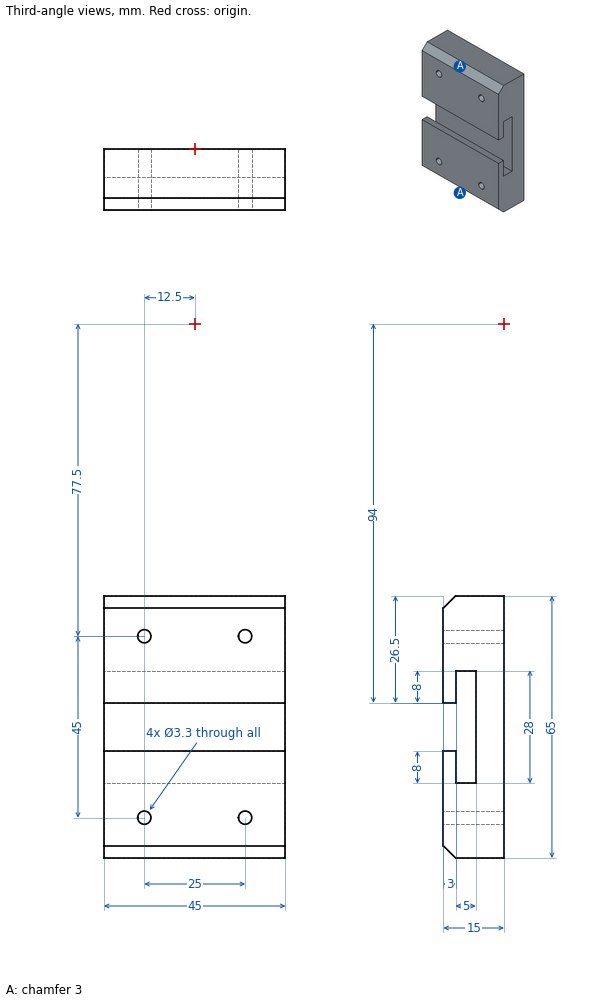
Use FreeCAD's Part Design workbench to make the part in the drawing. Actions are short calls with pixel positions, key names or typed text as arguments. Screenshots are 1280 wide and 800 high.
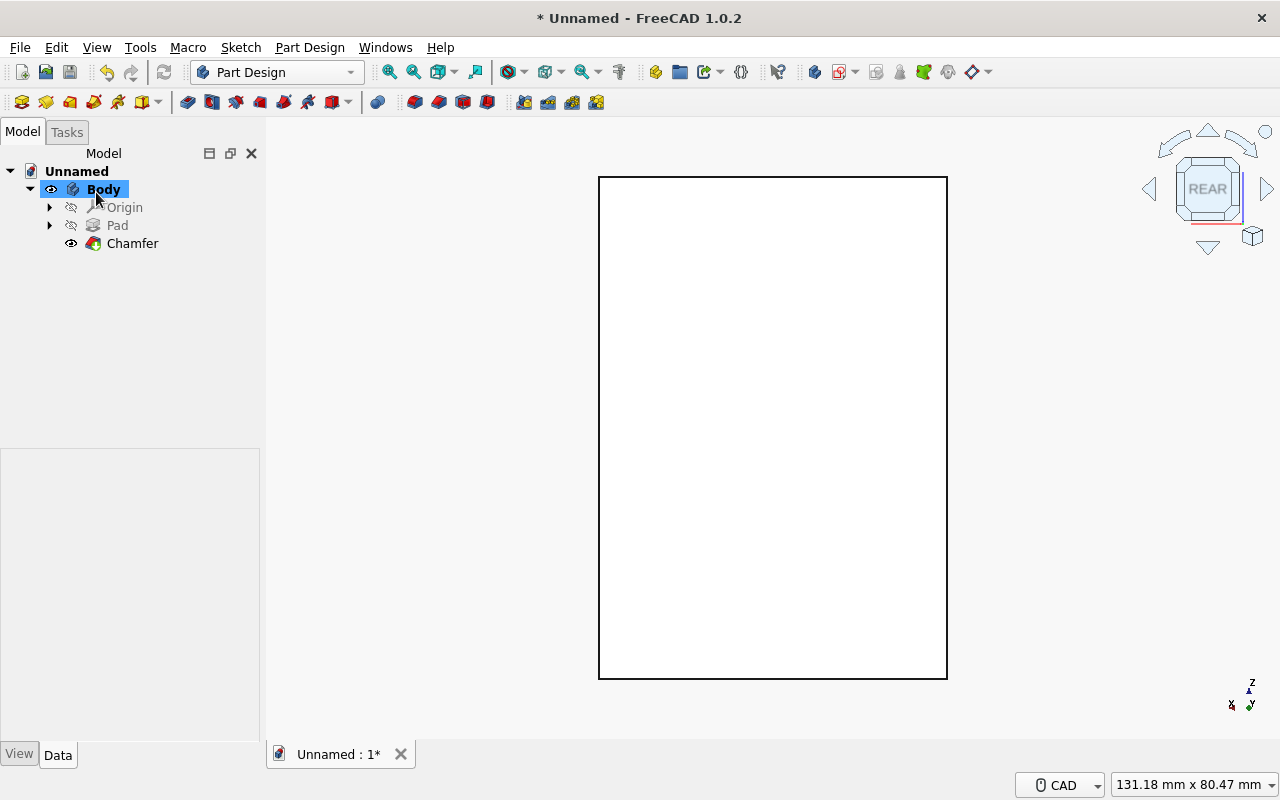
click(773, 499)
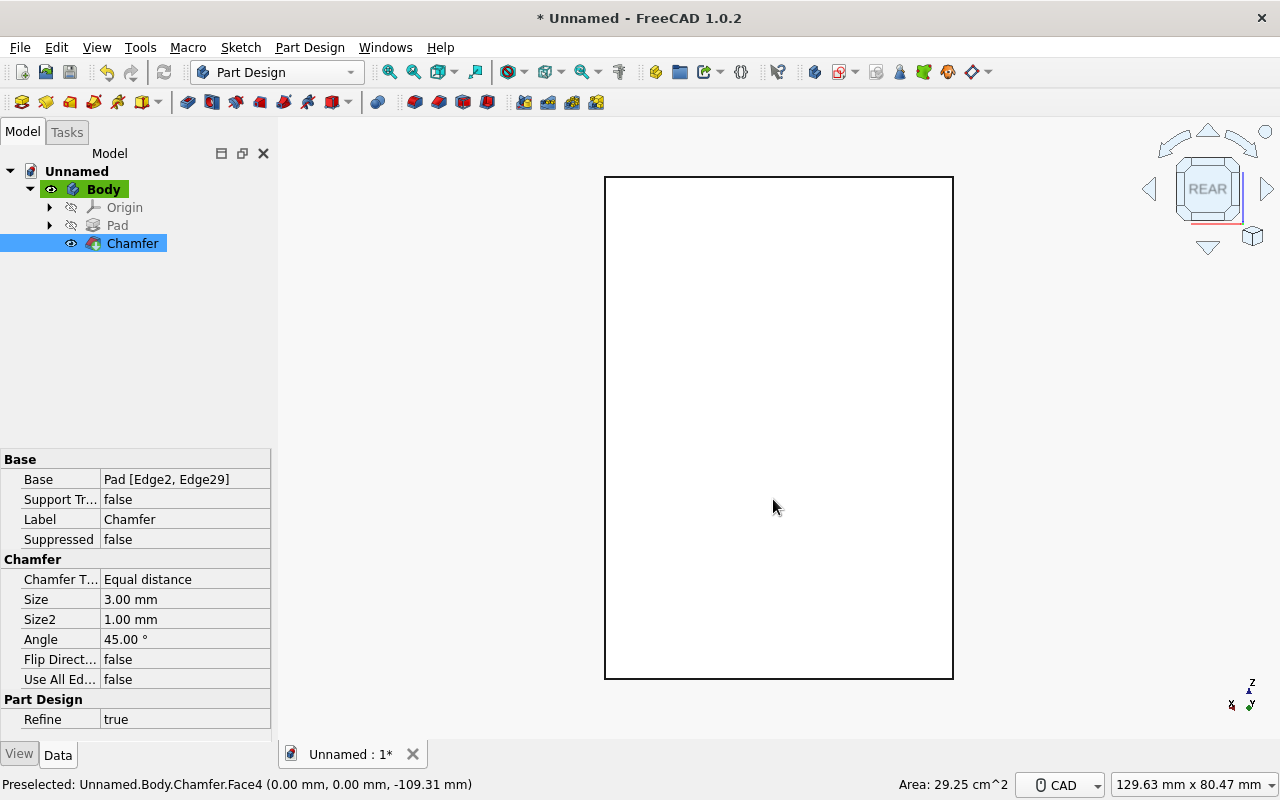
click(840, 72)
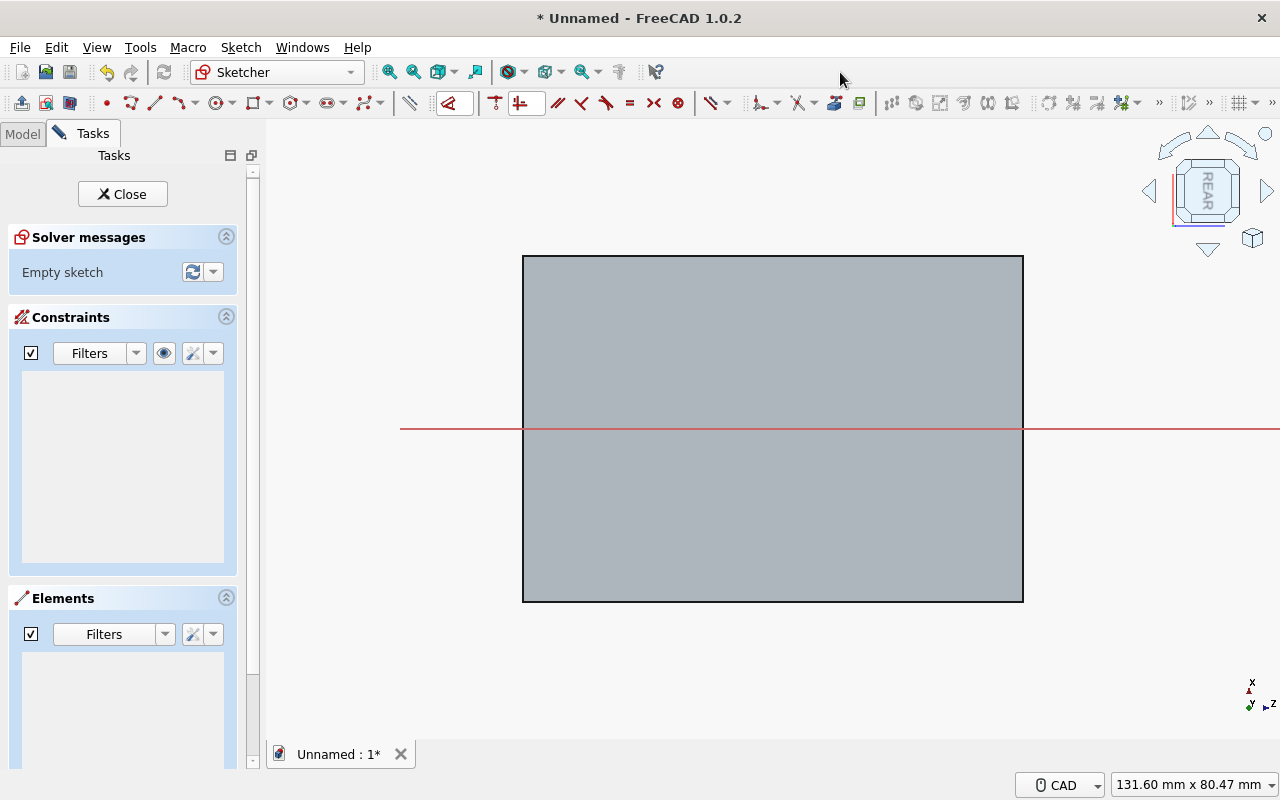
scroll(912, 429, up, 2)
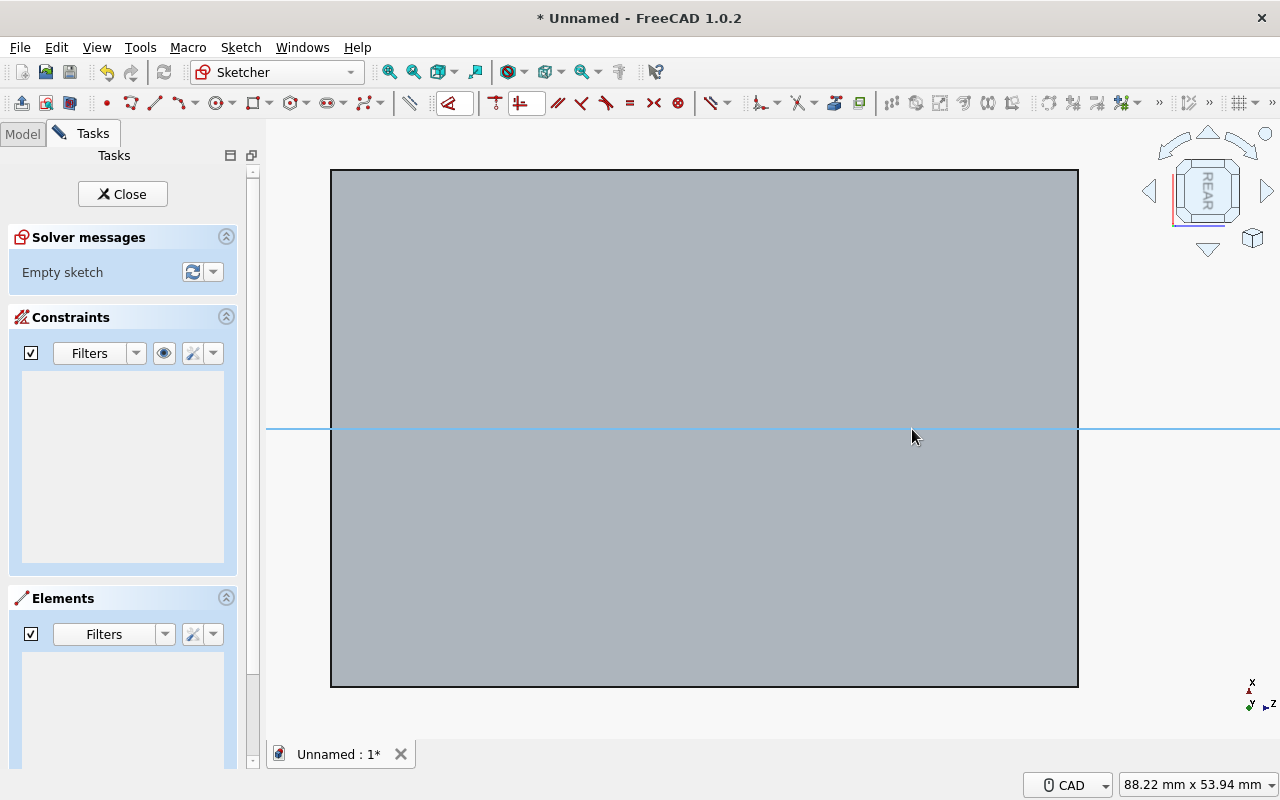
click(216, 104)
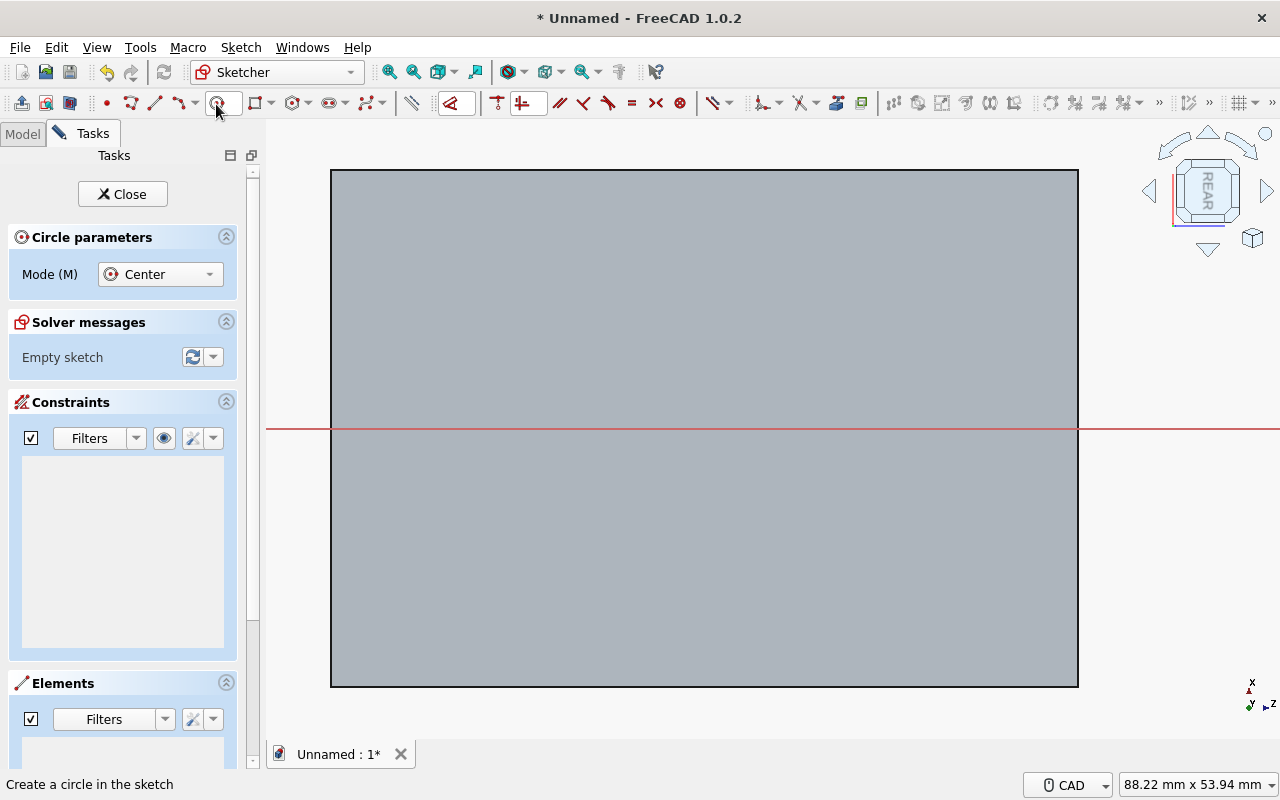
click(446, 572)
move(459, 559)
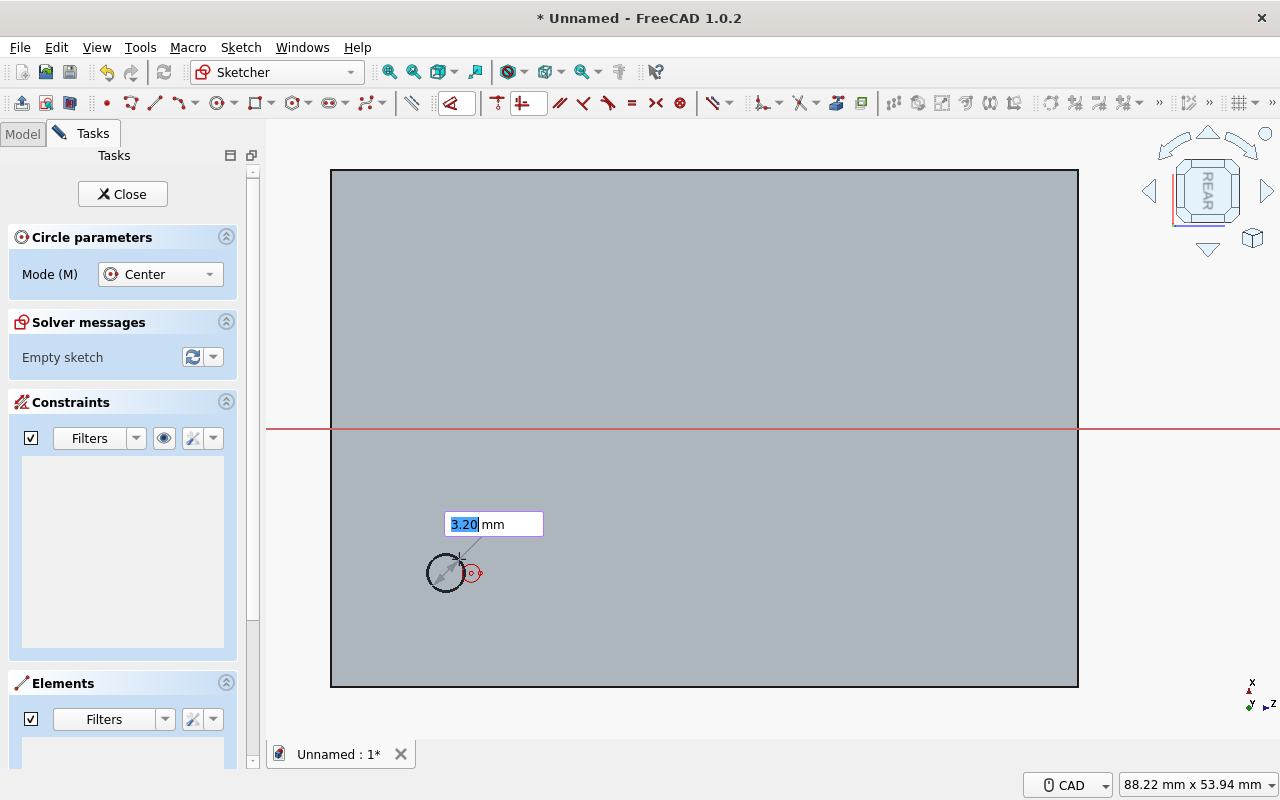
text(3.3)
key(Return)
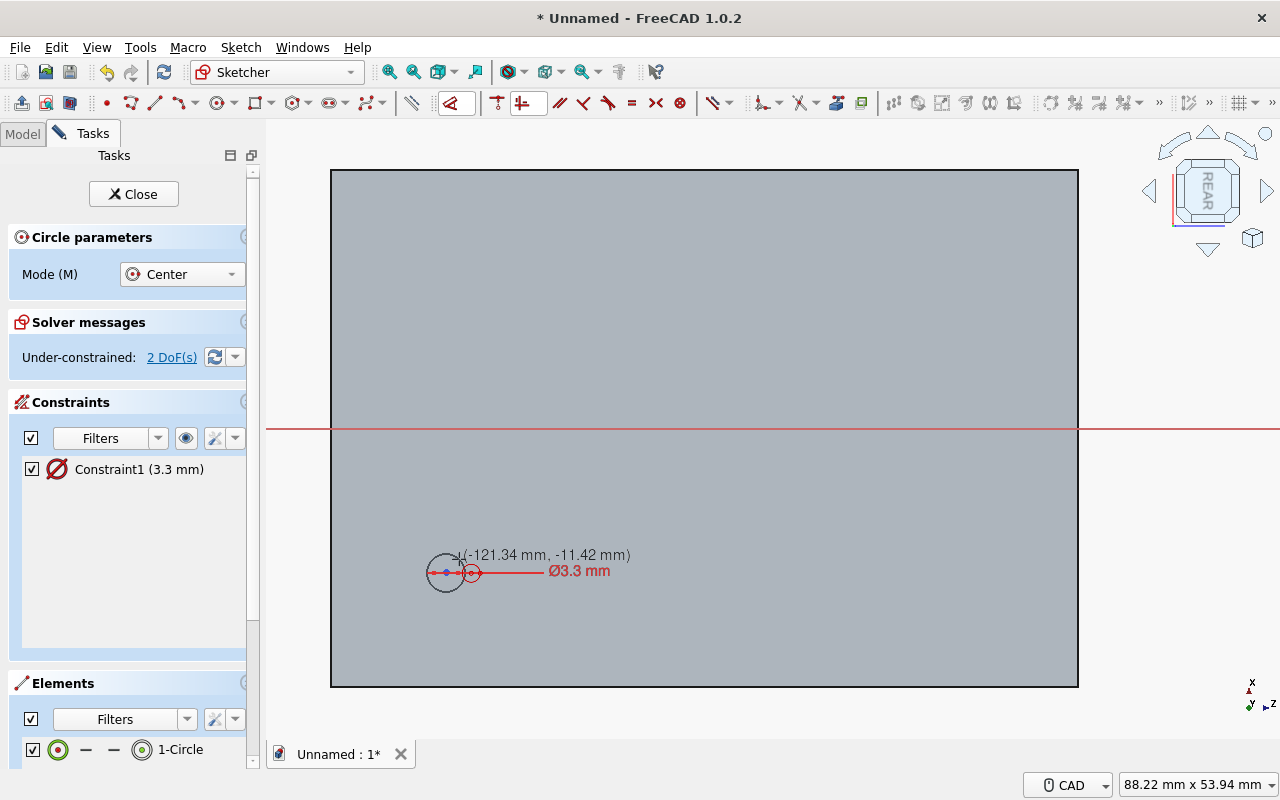
click(446, 285)
move(459, 272)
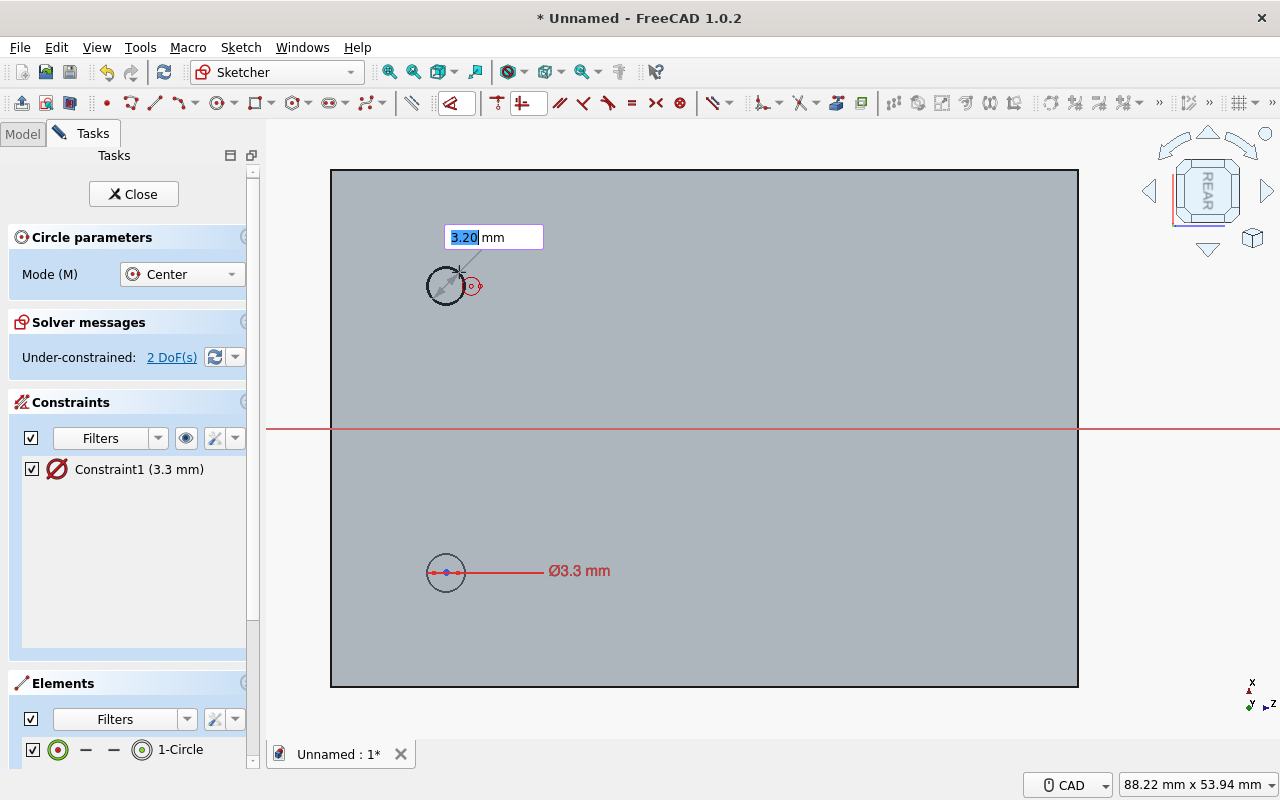
text(3.3)
key(Return)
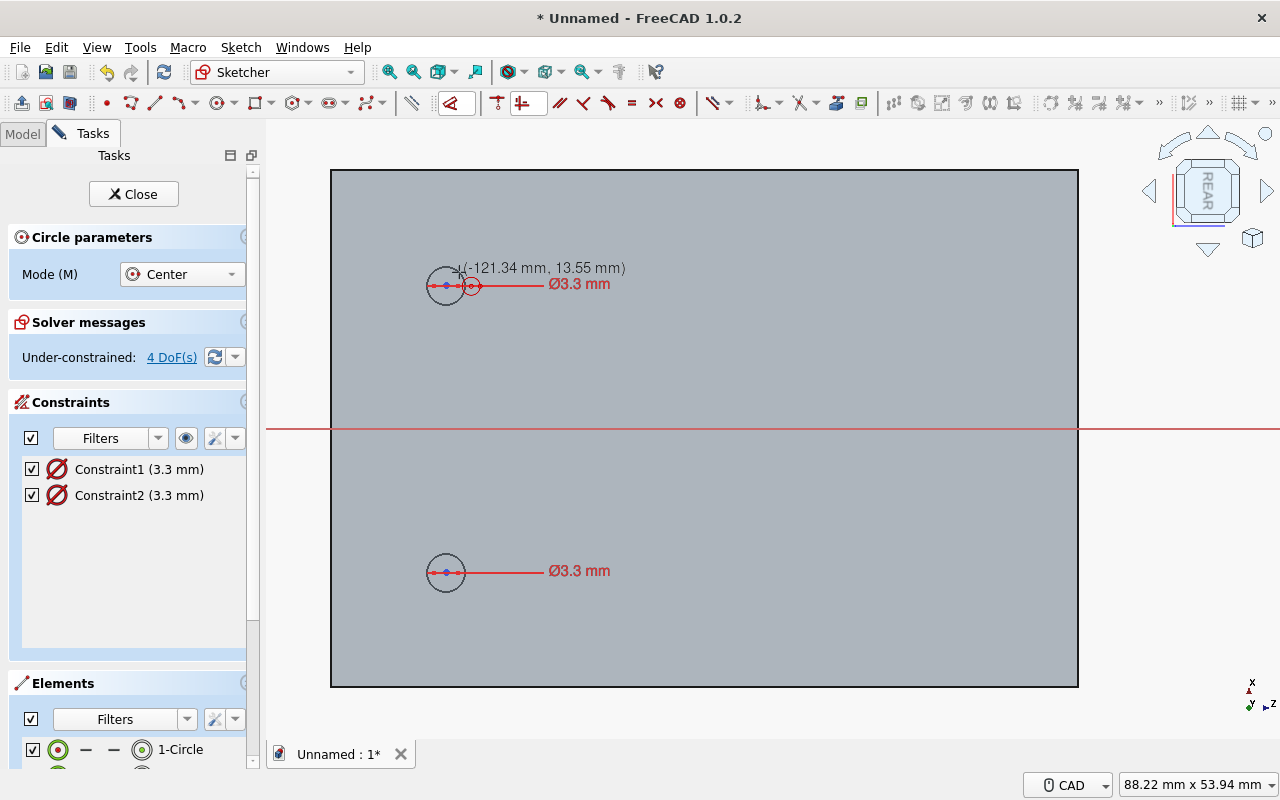
click(963, 572)
move(976, 559)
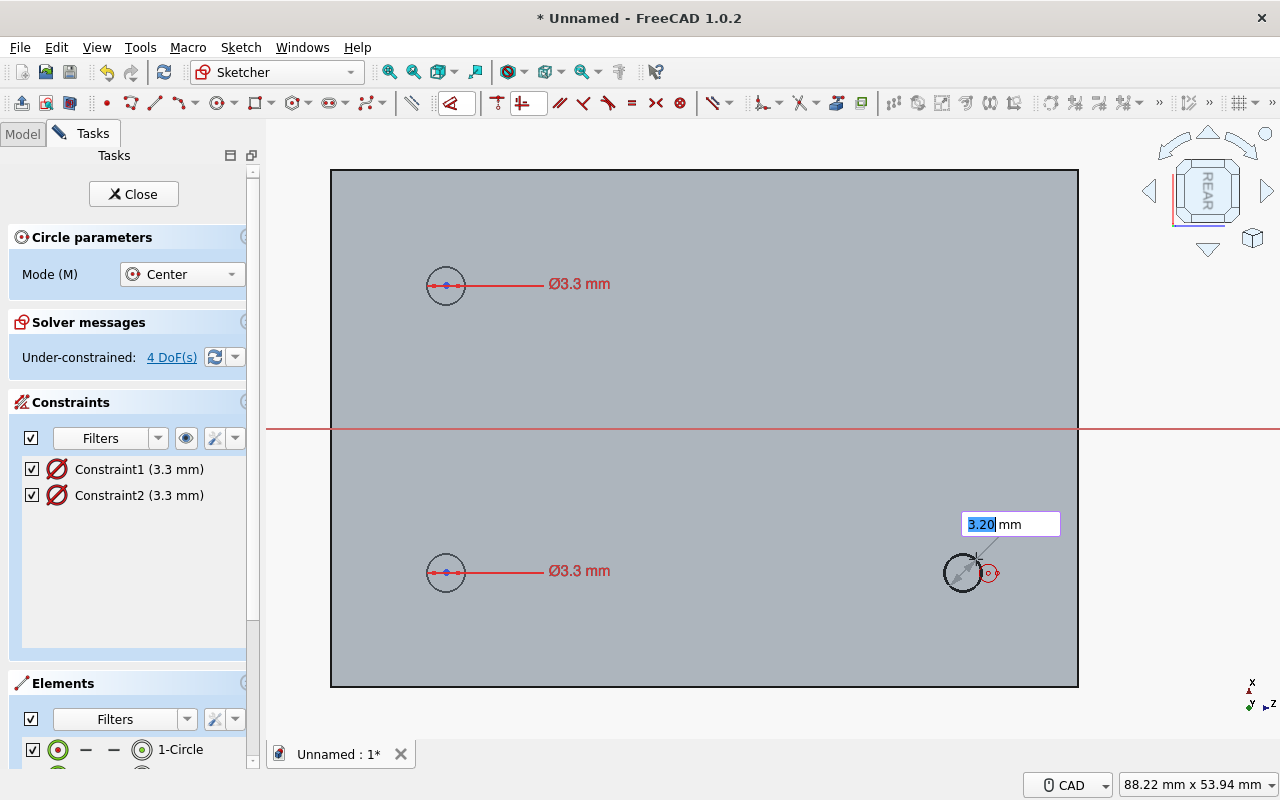
text(3.3)
key(Return)